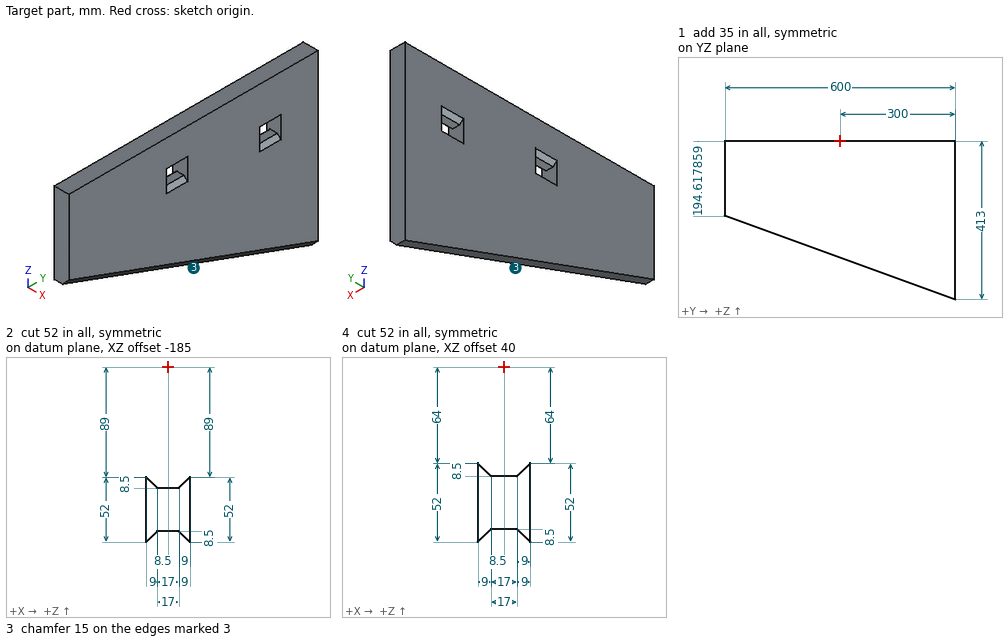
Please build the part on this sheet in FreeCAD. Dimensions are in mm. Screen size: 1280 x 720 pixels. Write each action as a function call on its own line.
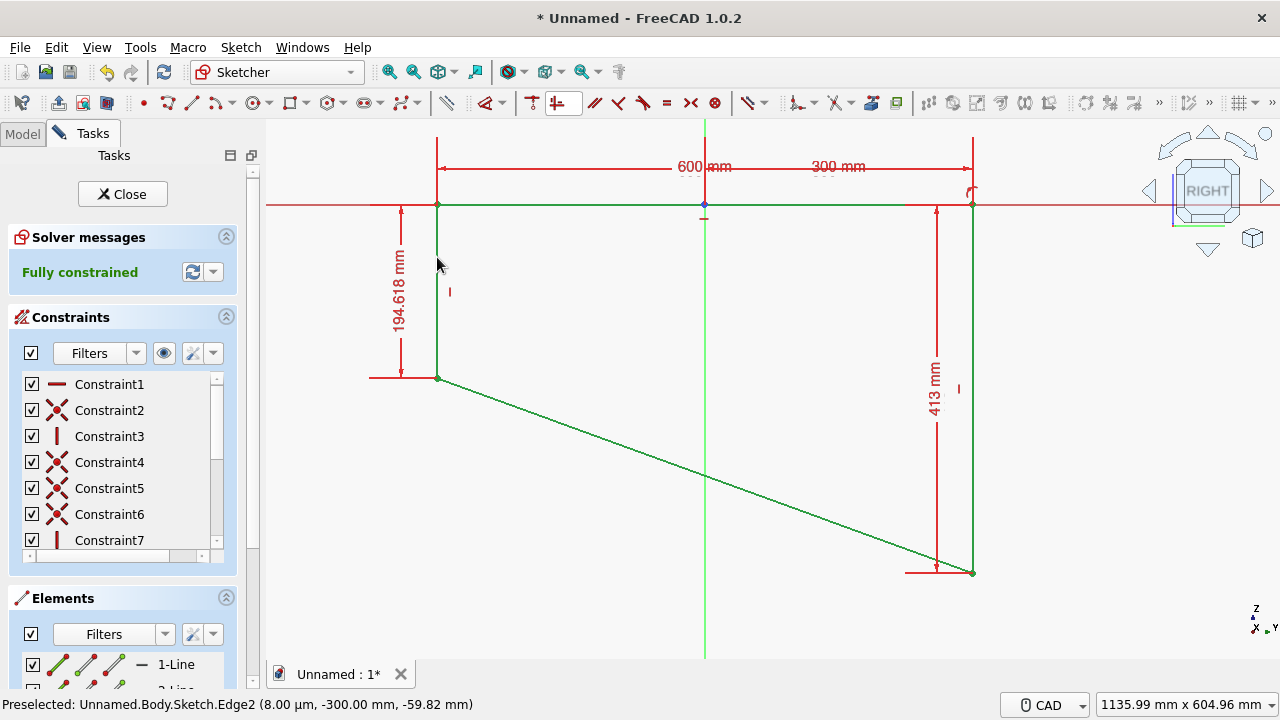
click(123, 194)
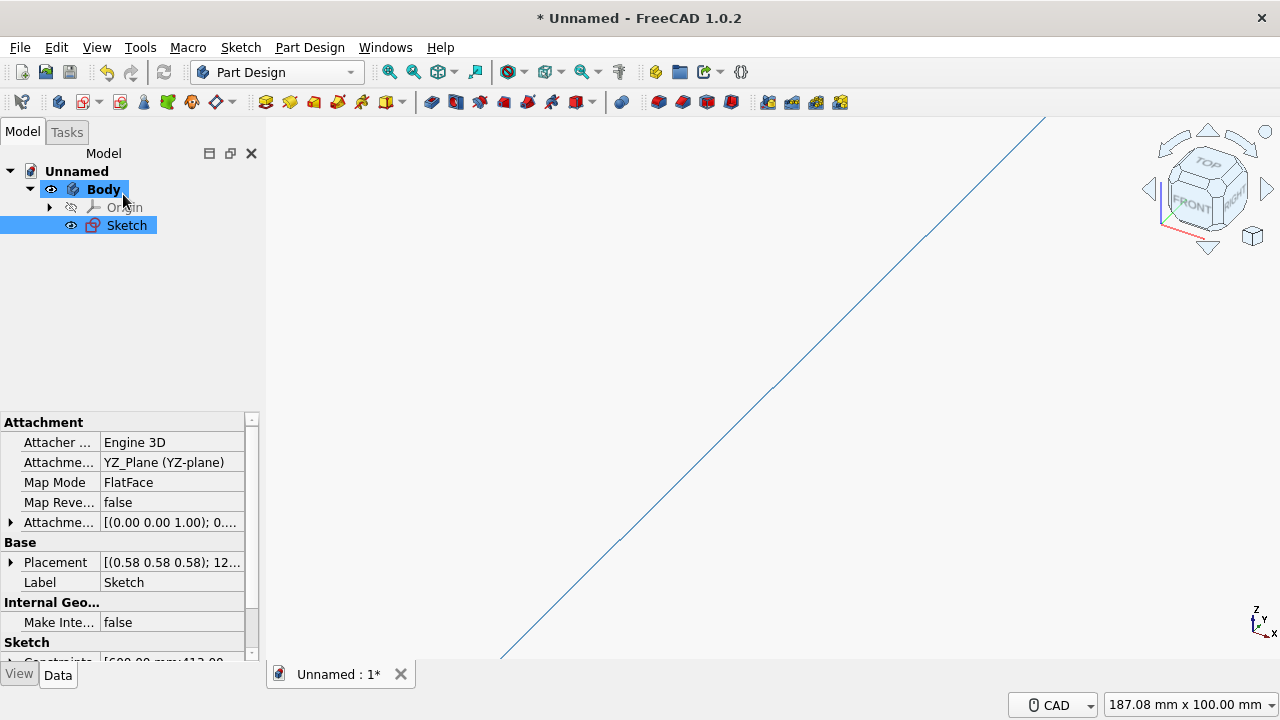
click(266, 102)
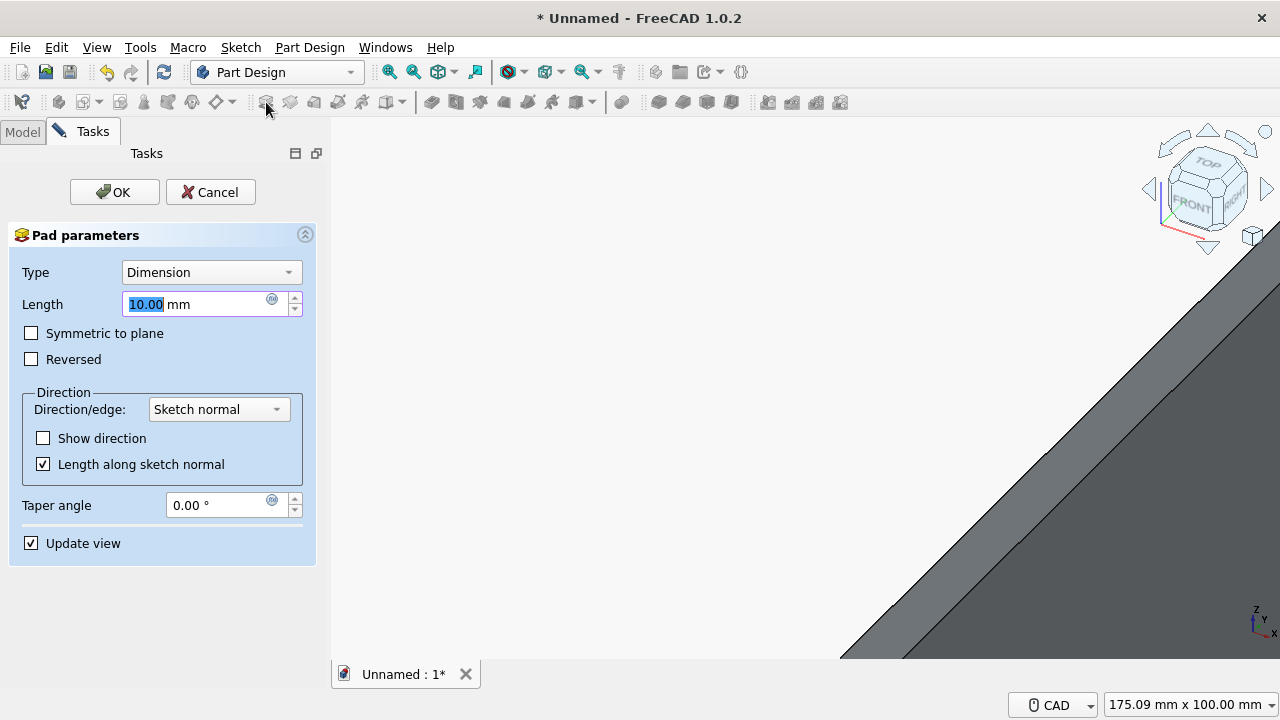
text(35)
key(Tab)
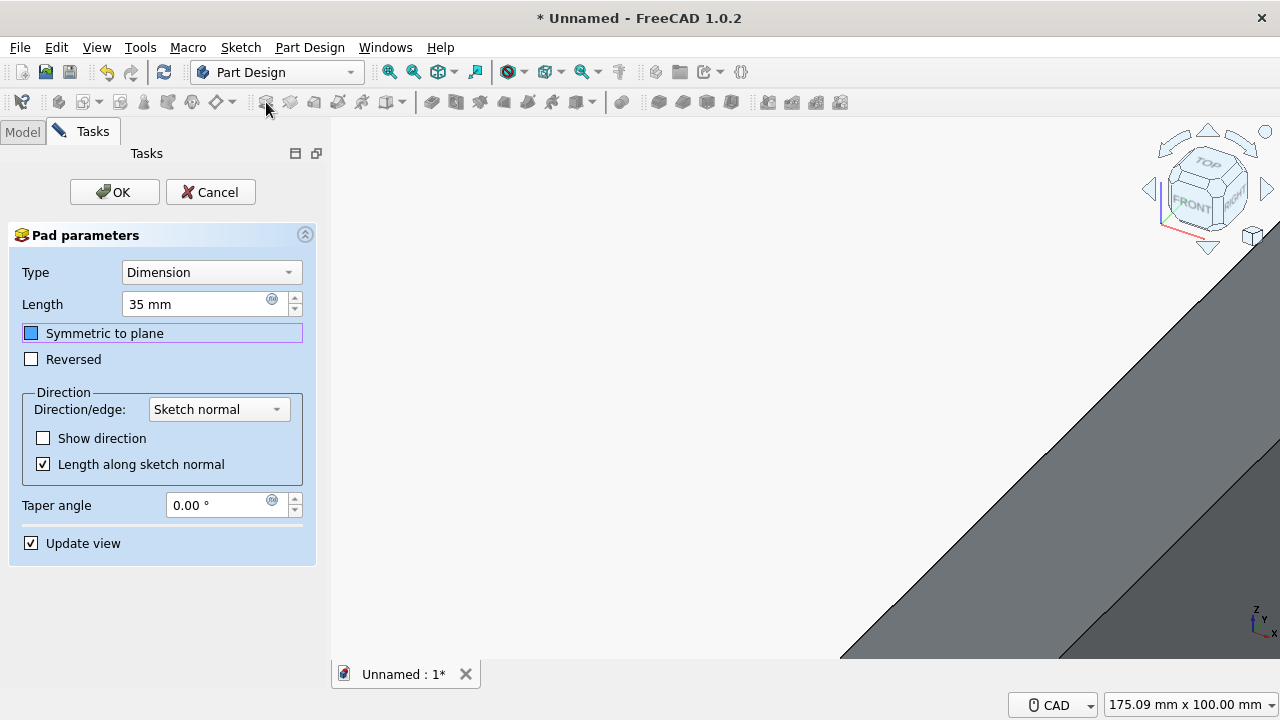
click(30, 333)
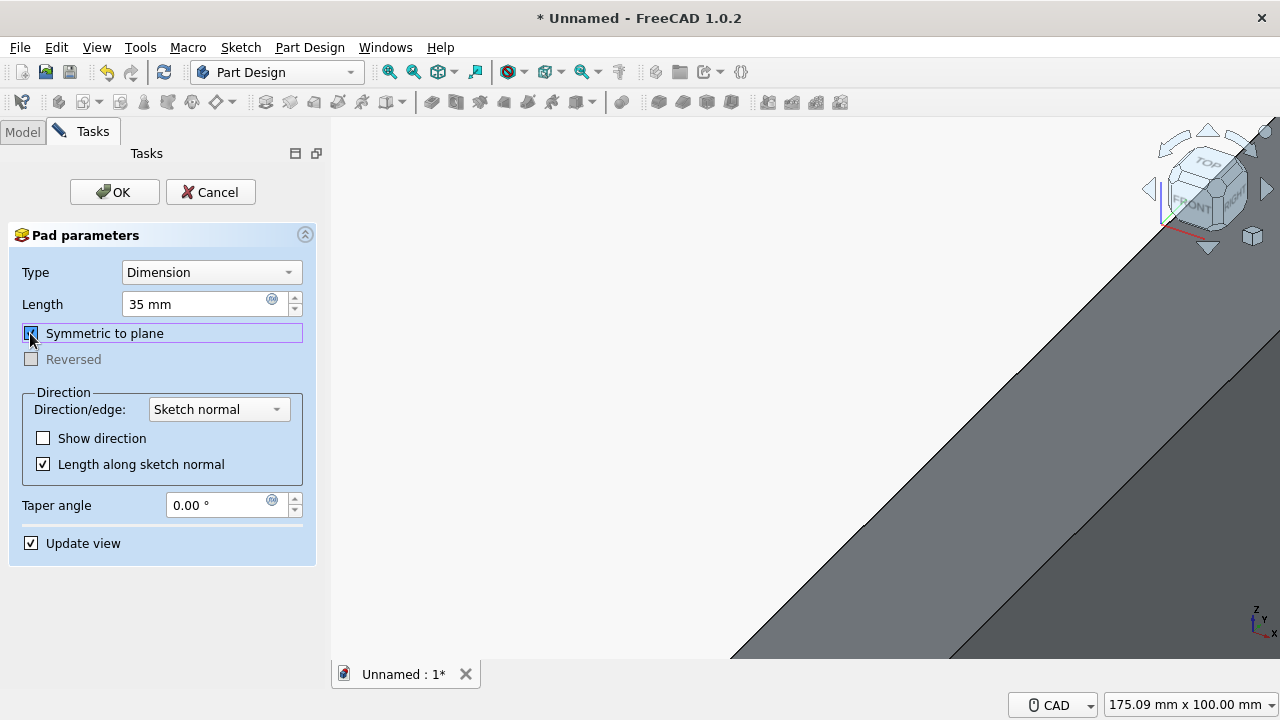
click(115, 192)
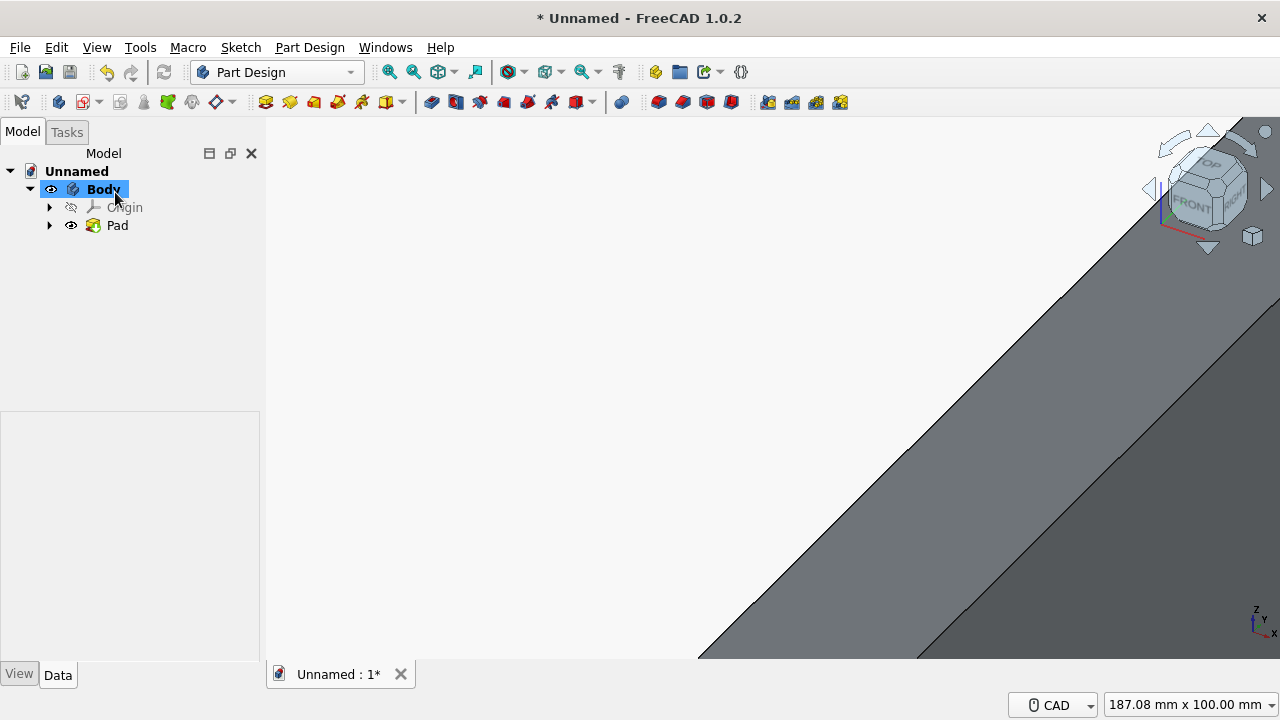
click(390, 72)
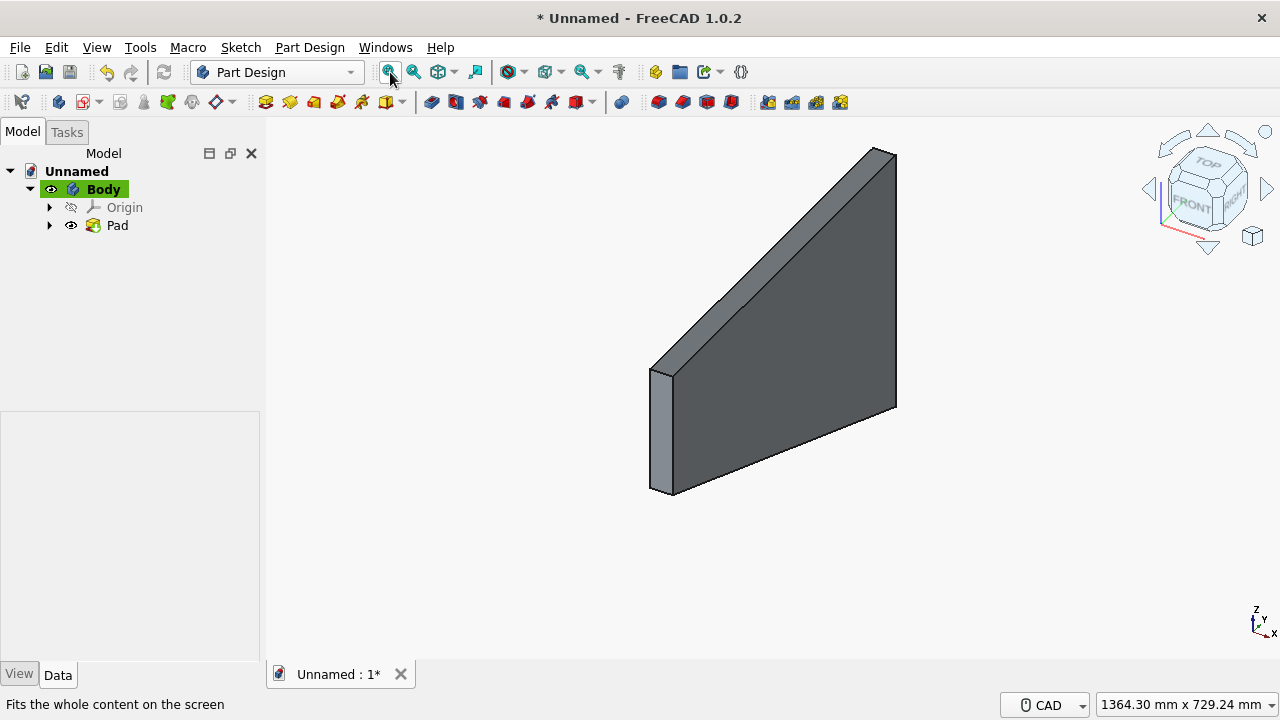
click(50, 207)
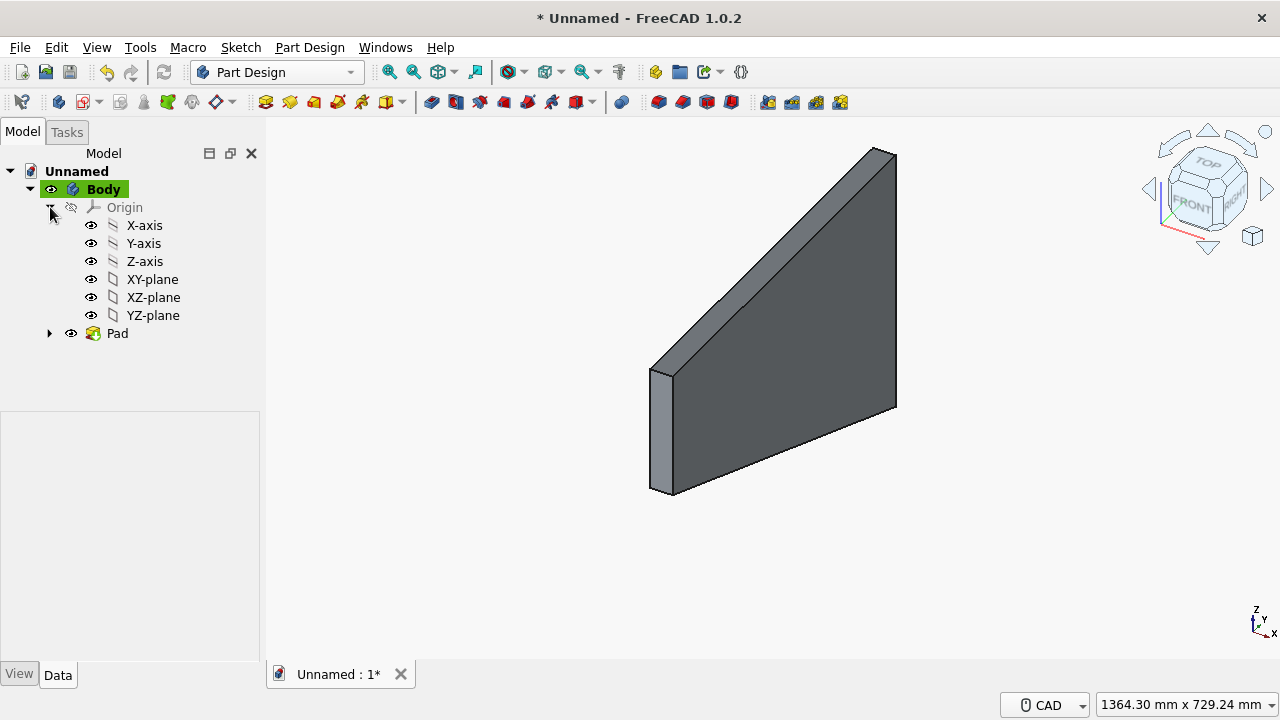
click(136, 297)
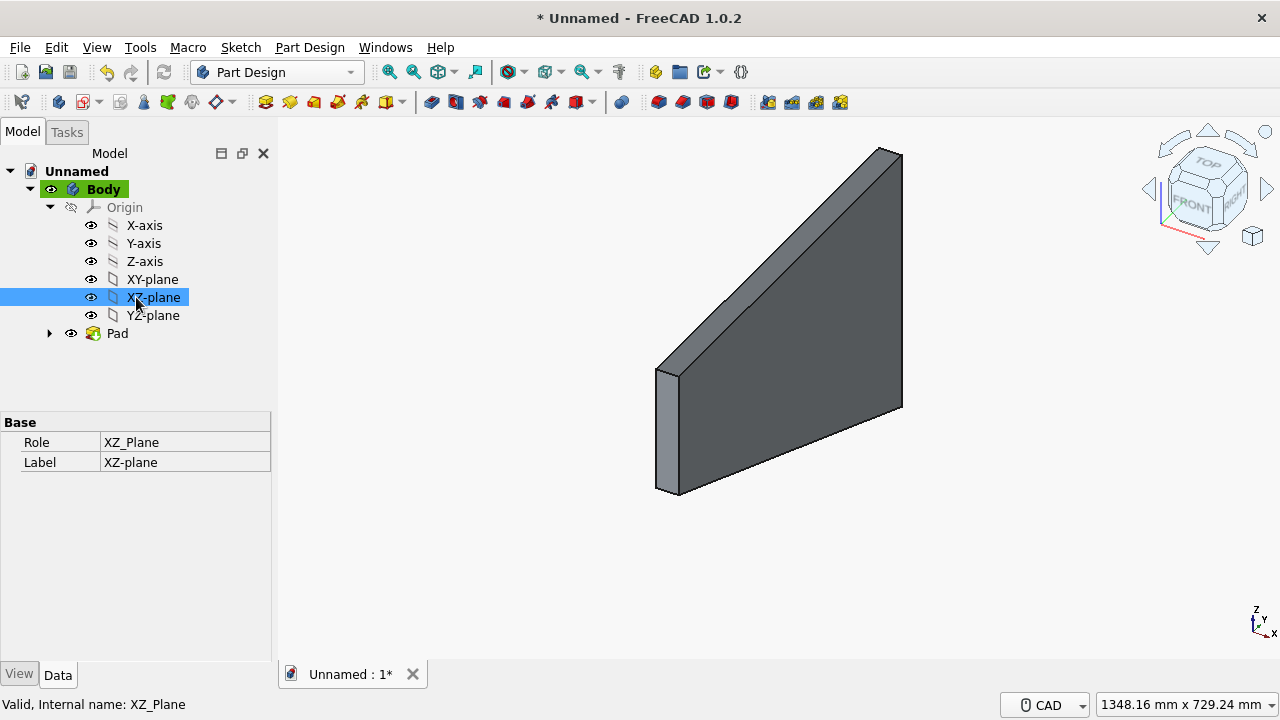
click(216, 102)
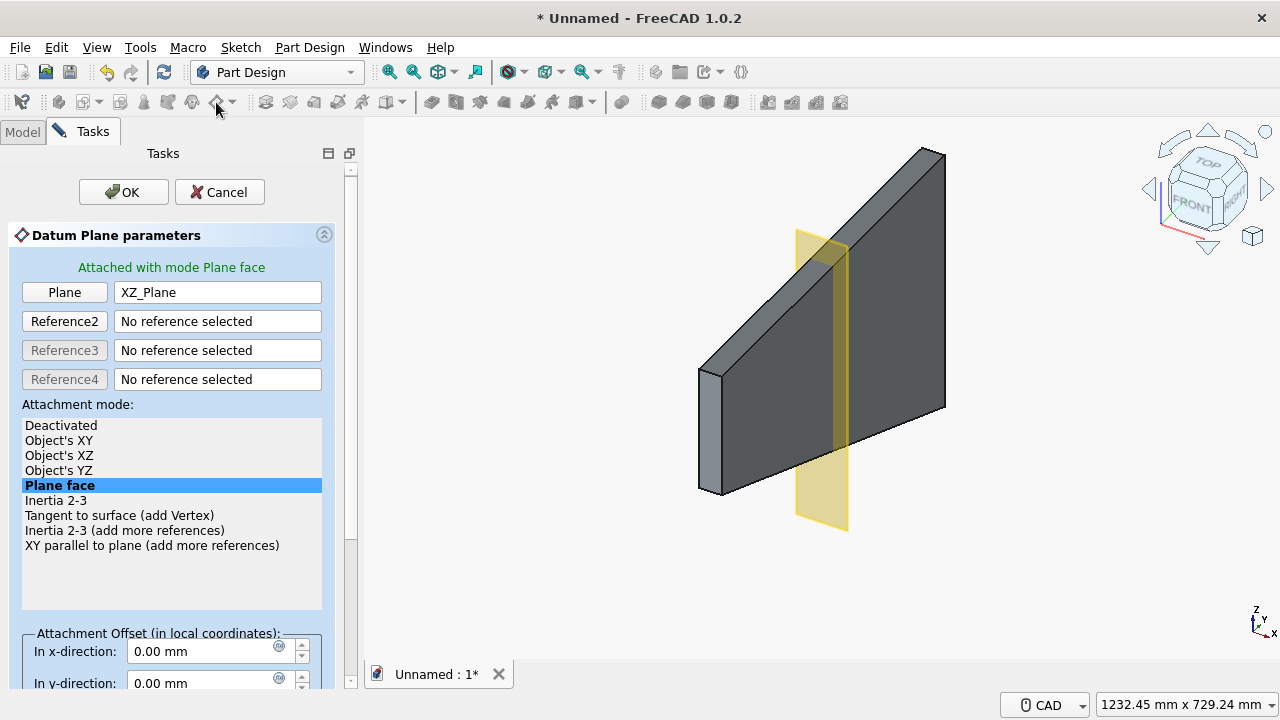
scroll(351, 426, down, 2)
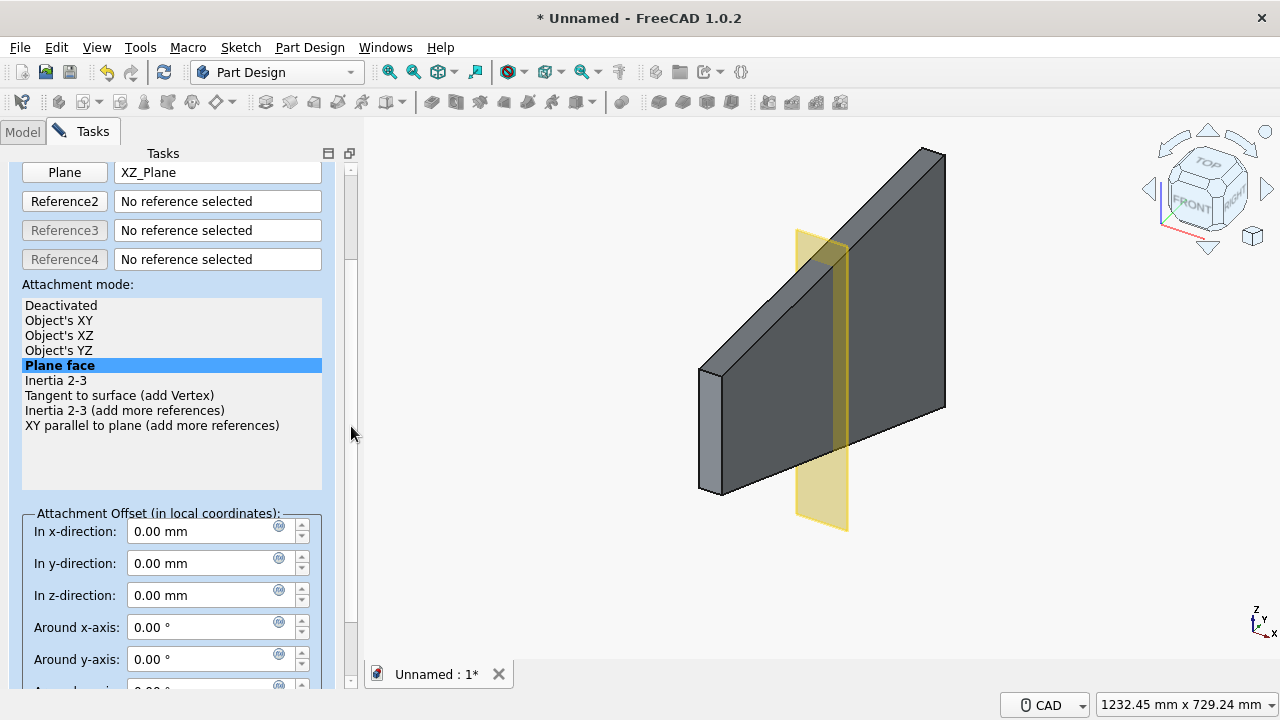
triple_click(210, 595)